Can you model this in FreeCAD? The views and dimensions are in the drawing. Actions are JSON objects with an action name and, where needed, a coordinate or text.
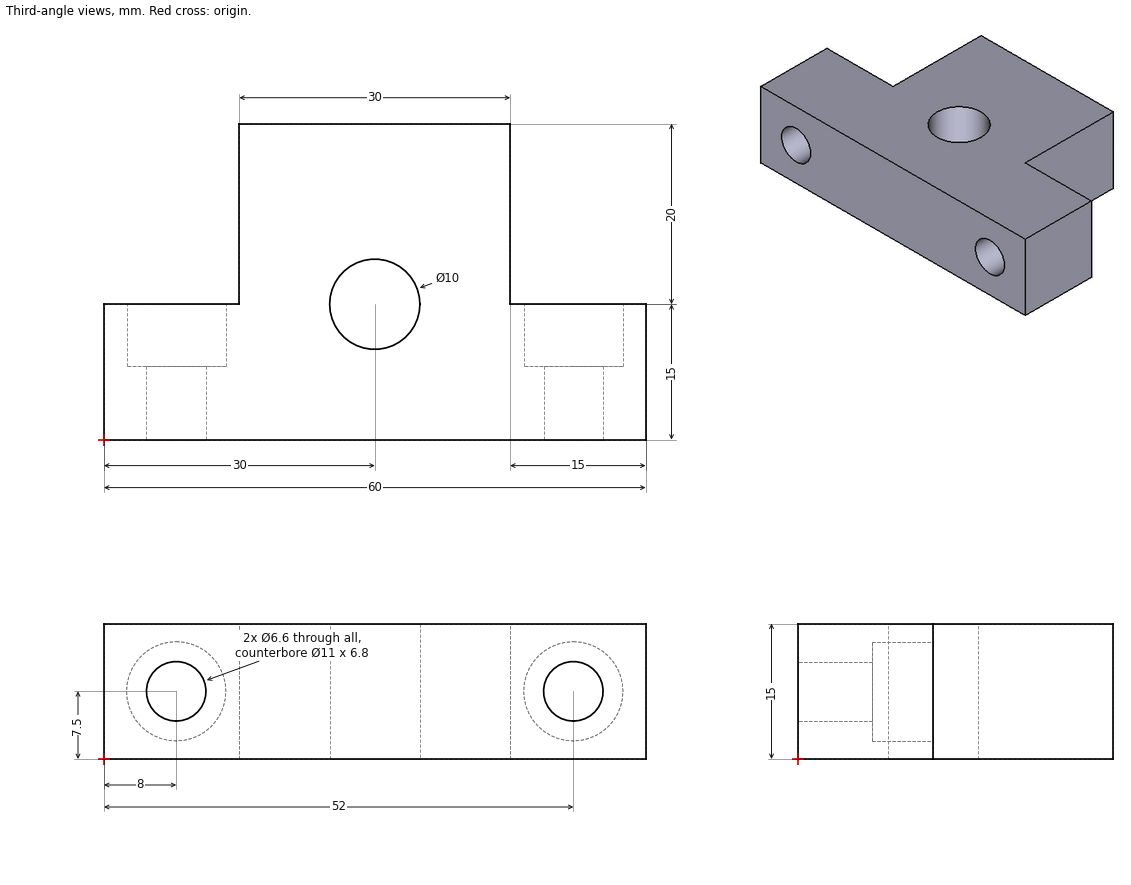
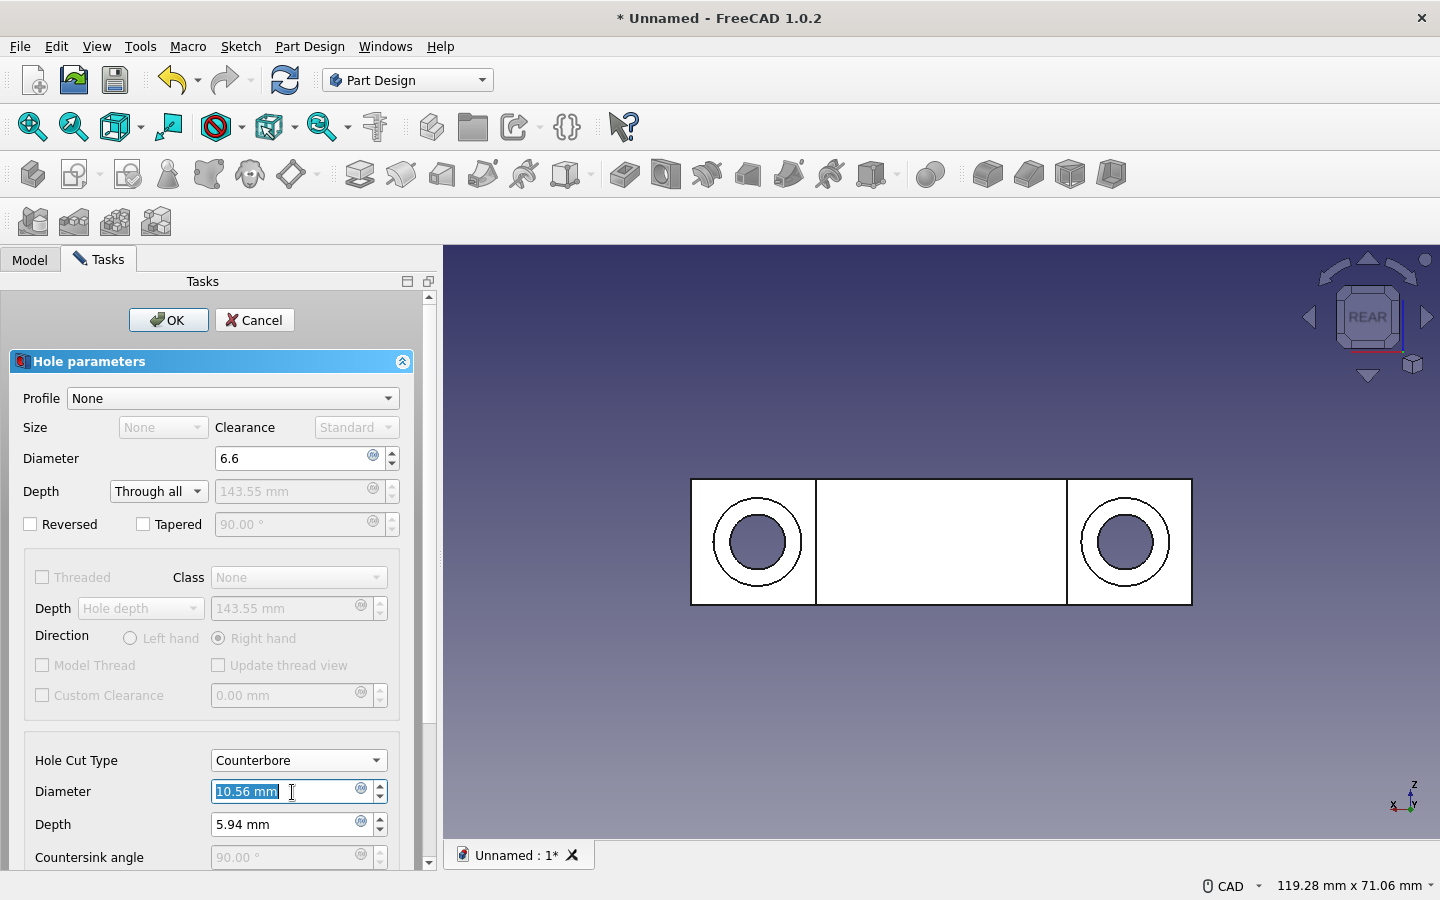
{"action": "type", "text": "11"}
{"action": "key", "text": "Tab"}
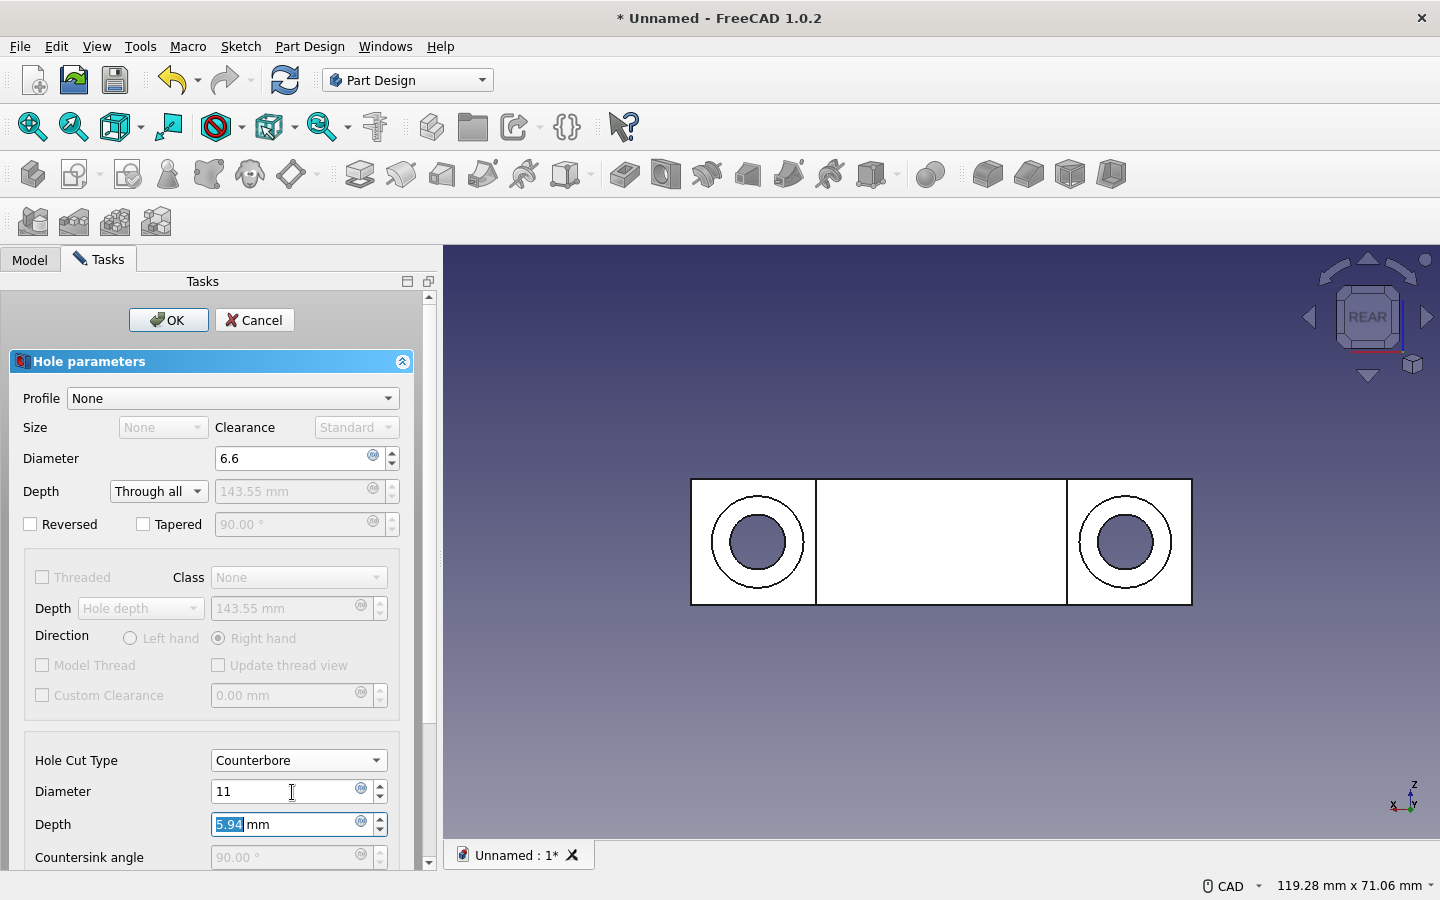
{"action": "type", "text": "6.8"}
{"action": "key", "text": "Tab"}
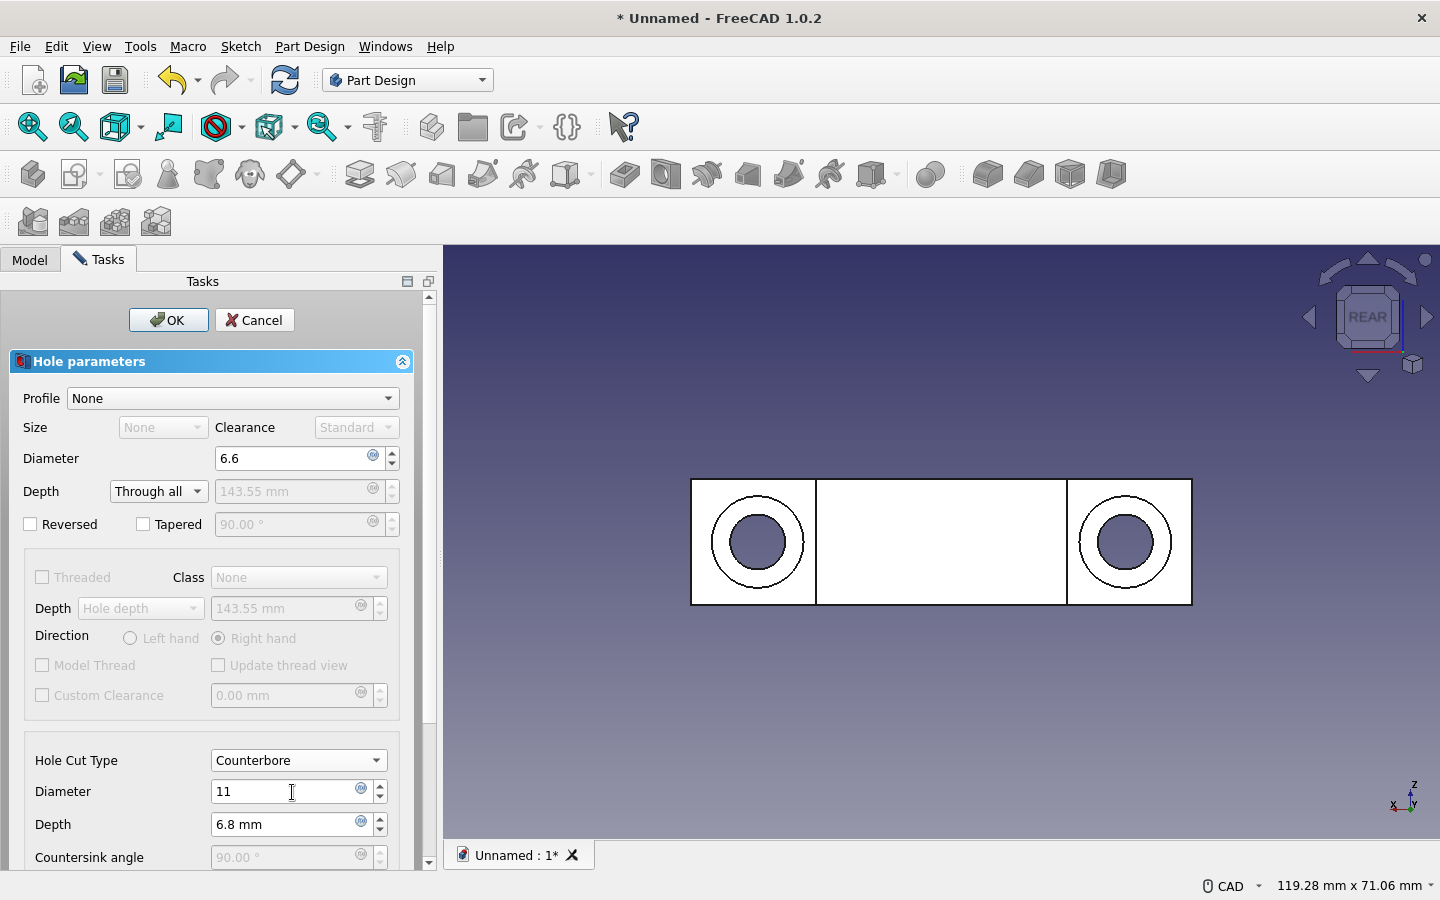
{"action": "left_click", "coordinate": [169, 320]}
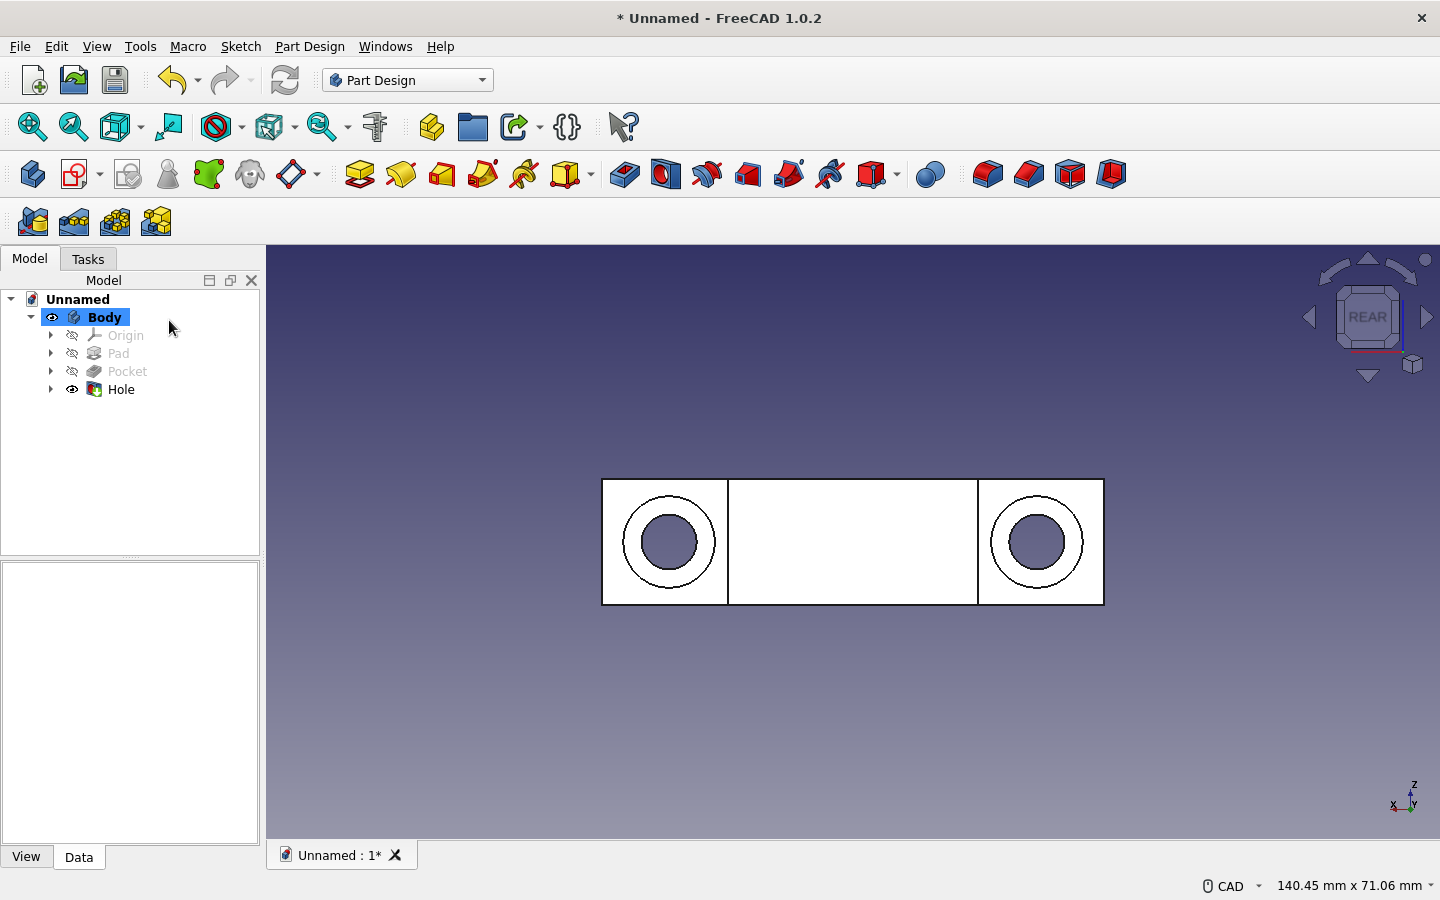
{"action": "key", "text": "0"}